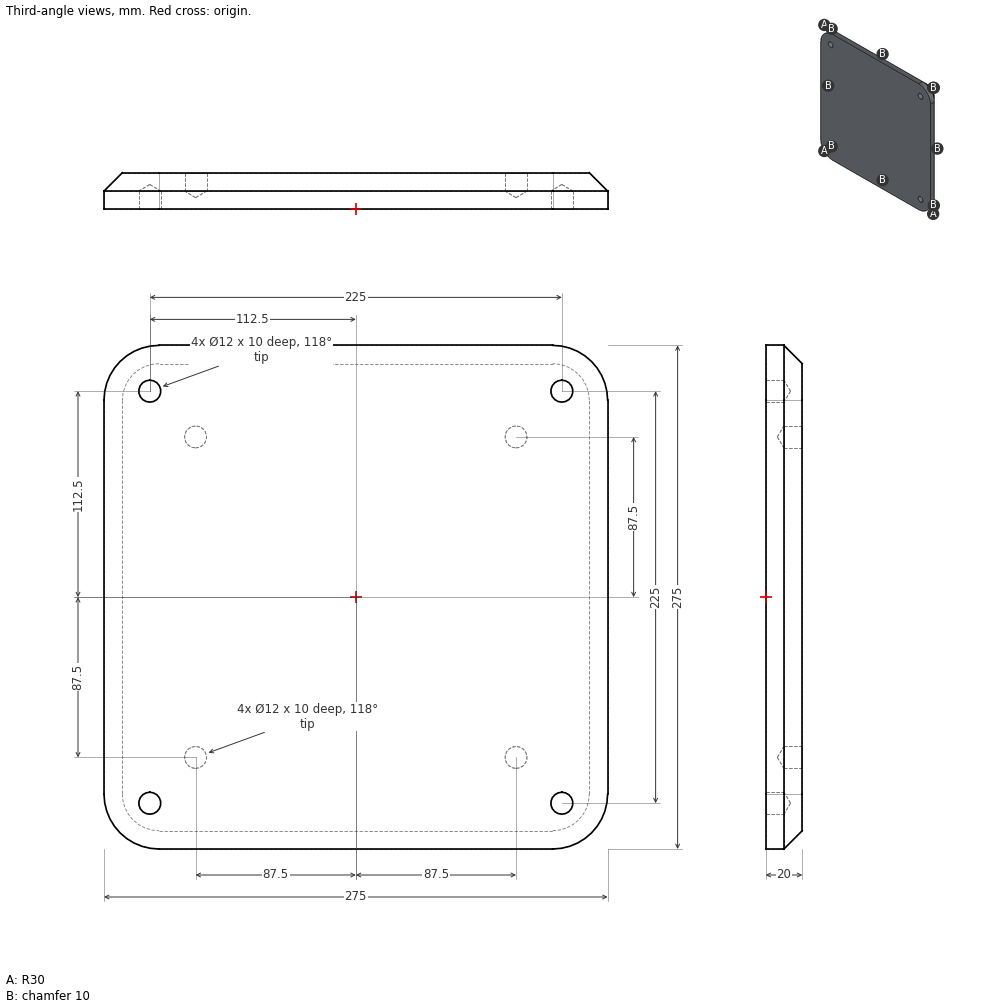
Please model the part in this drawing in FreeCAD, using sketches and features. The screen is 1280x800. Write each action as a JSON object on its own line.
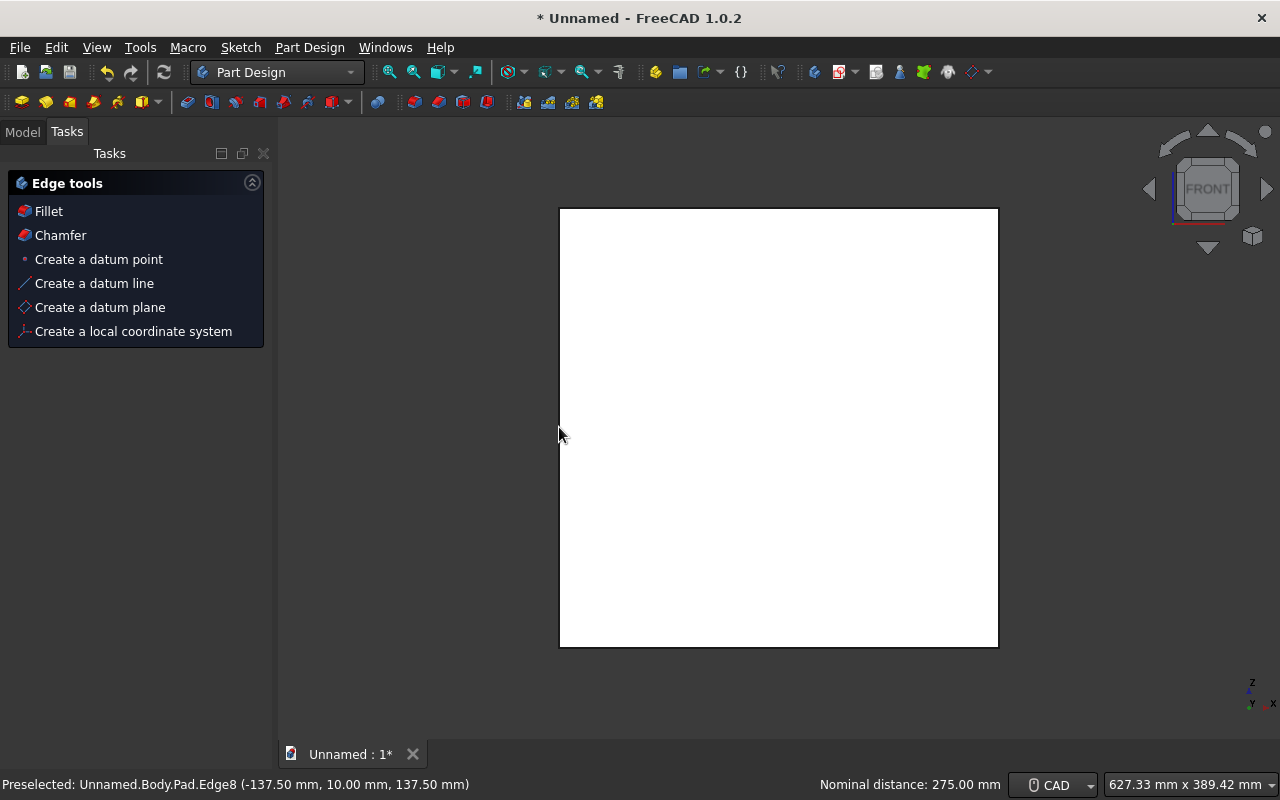
{"action": "key", "text": "3"}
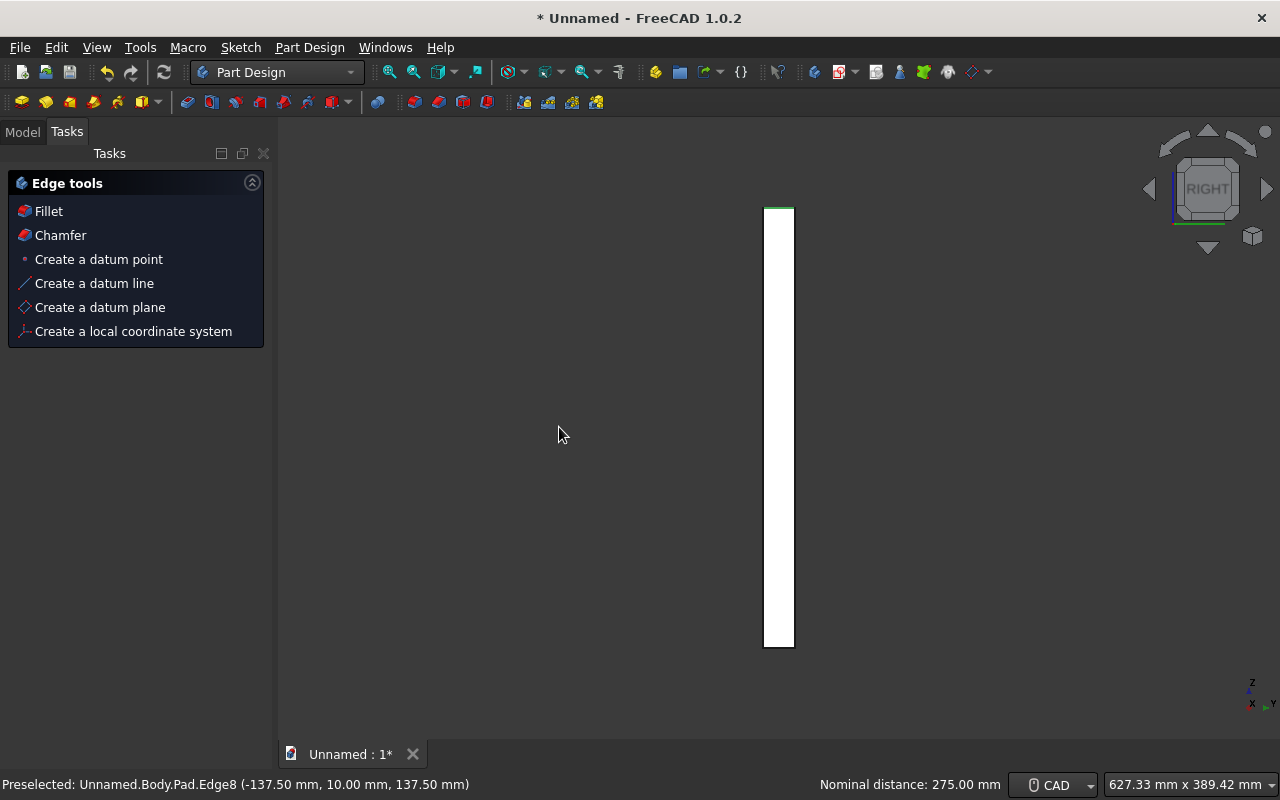
{"action": "left_click", "coordinate": [779, 647], "text": "ctrl"}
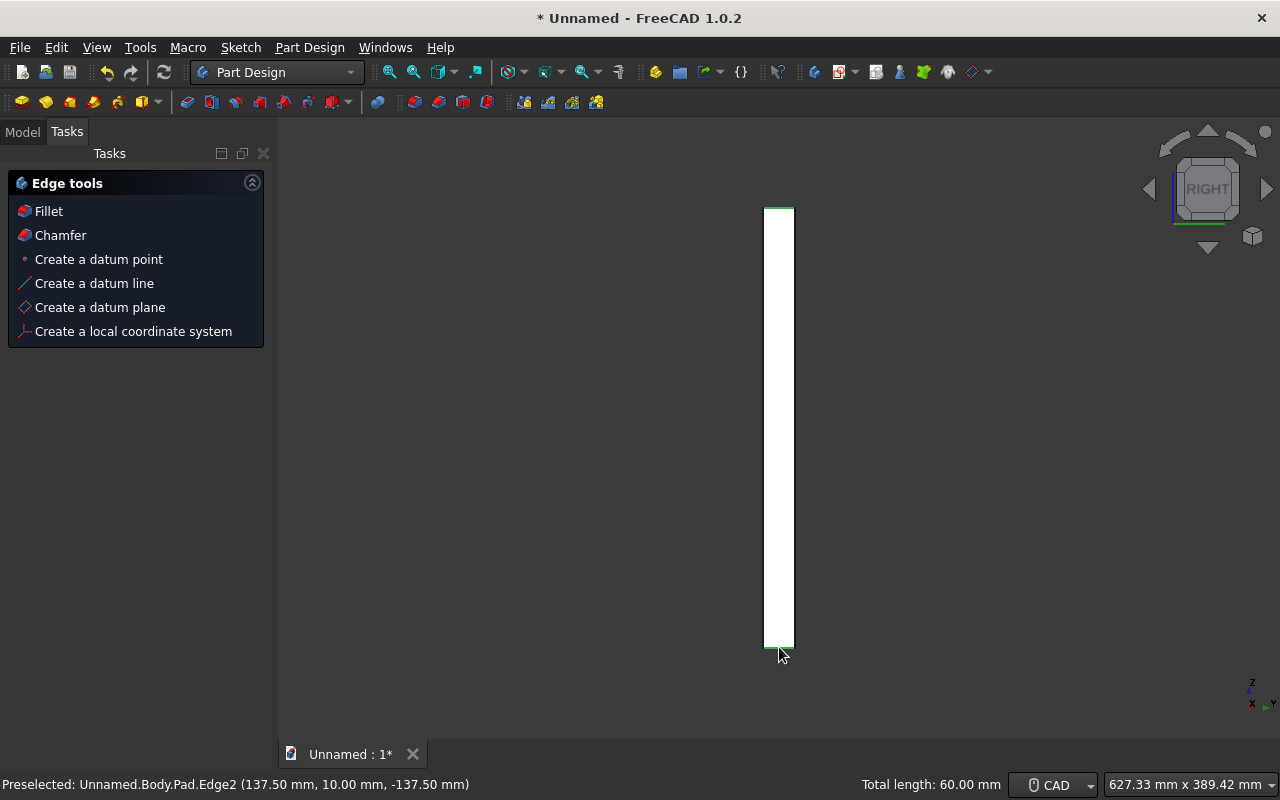
{"action": "key", "text": "5"}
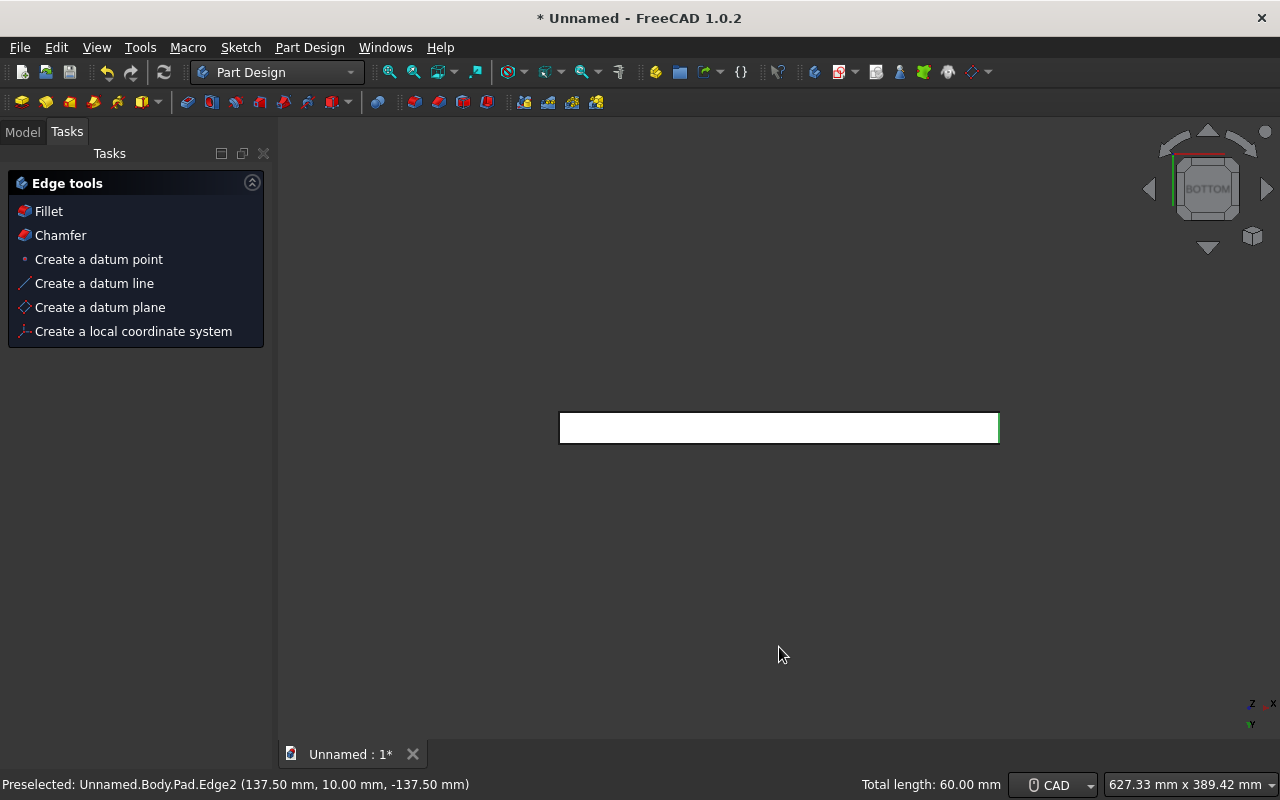
{"action": "key", "text": "v f"}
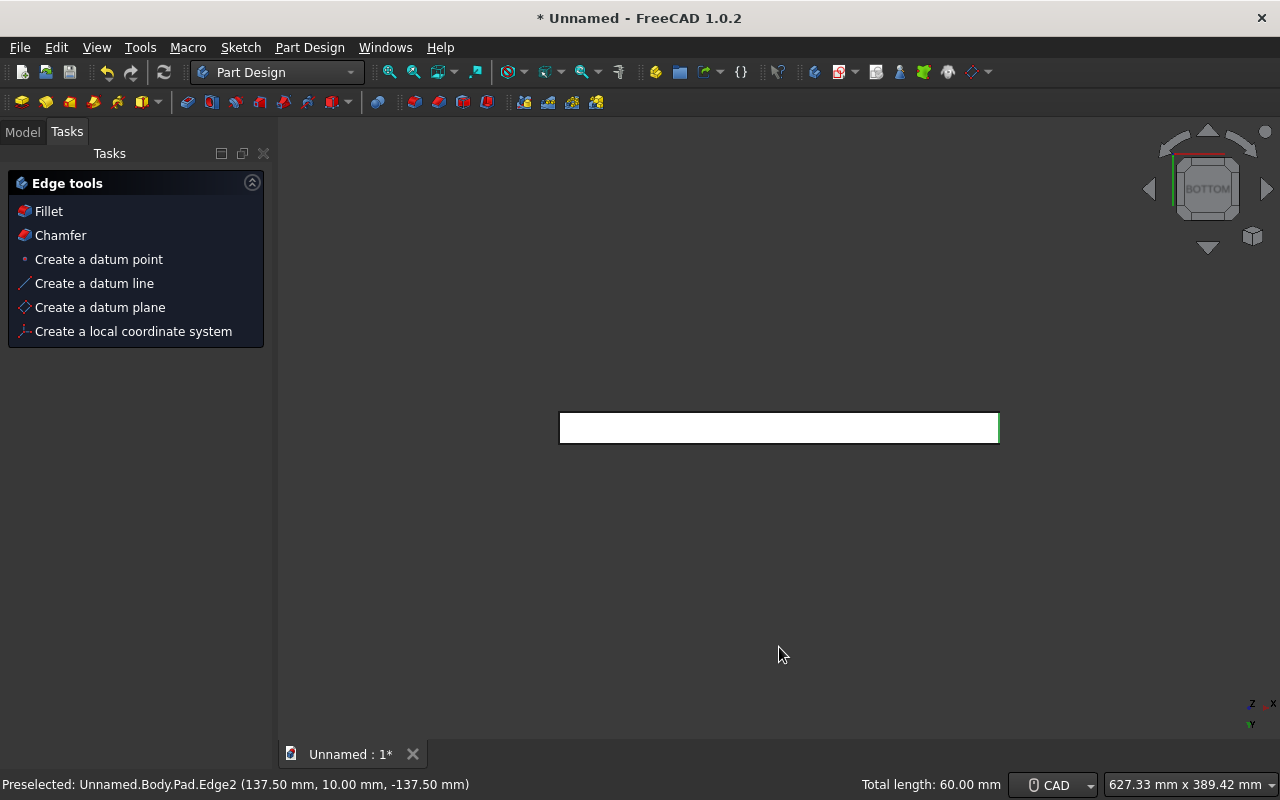
{"action": "left_click", "coordinate": [559, 427], "text": "ctrl"}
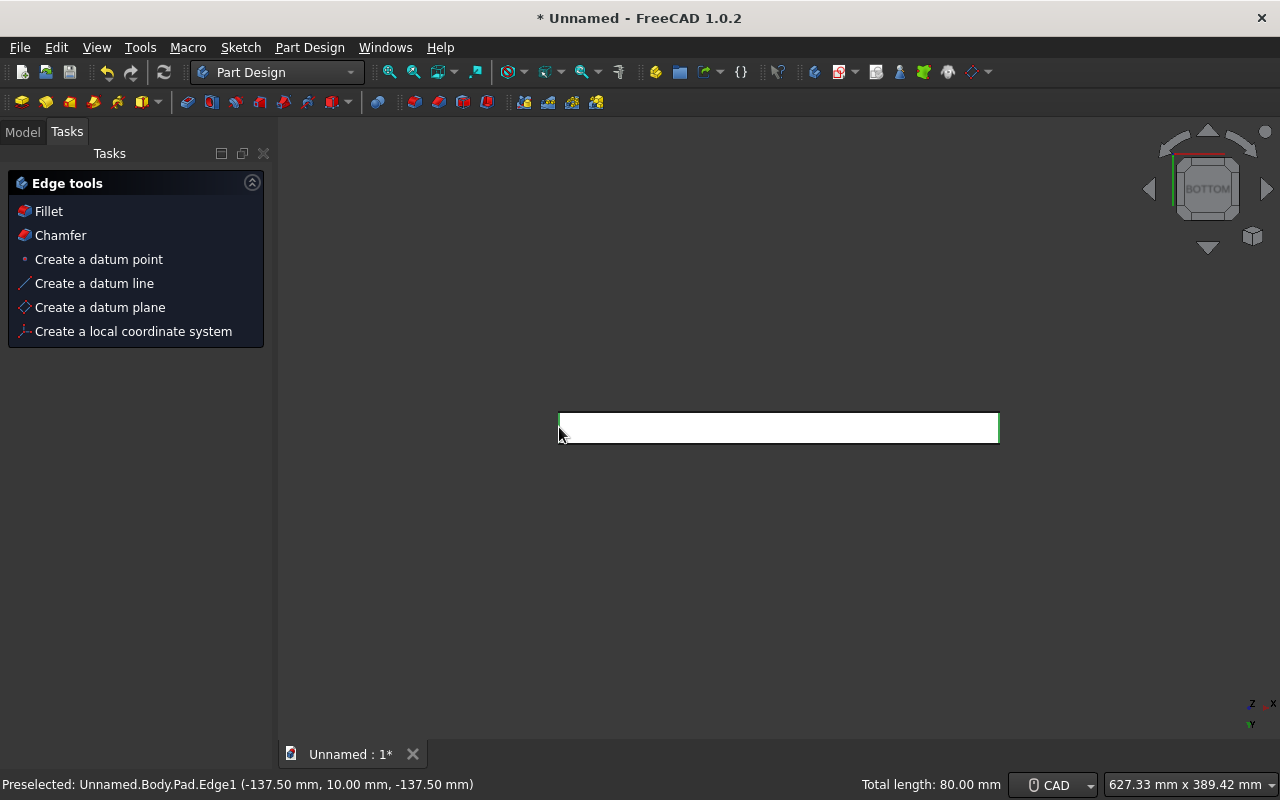
{"action": "left_click", "coordinate": [416, 102]}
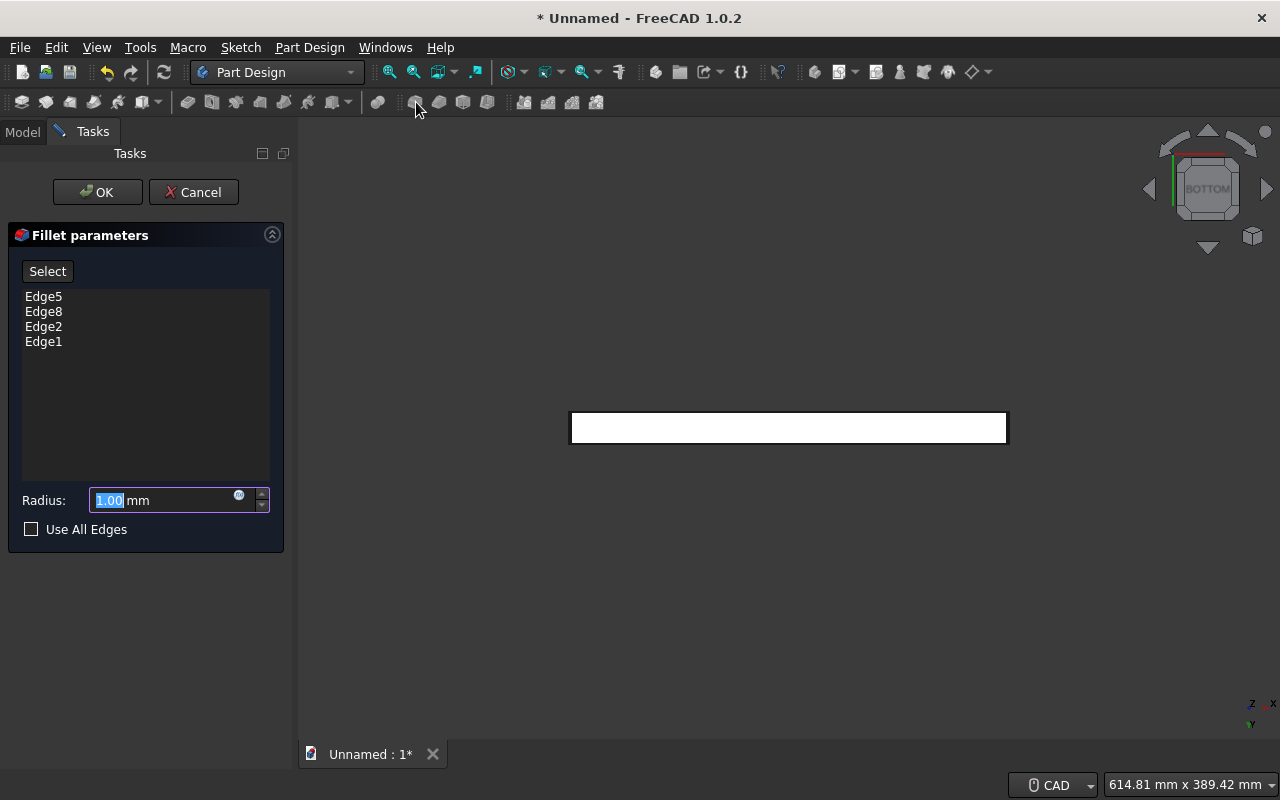
{"action": "type", "text": "30"}
{"action": "key", "text": "Tab"}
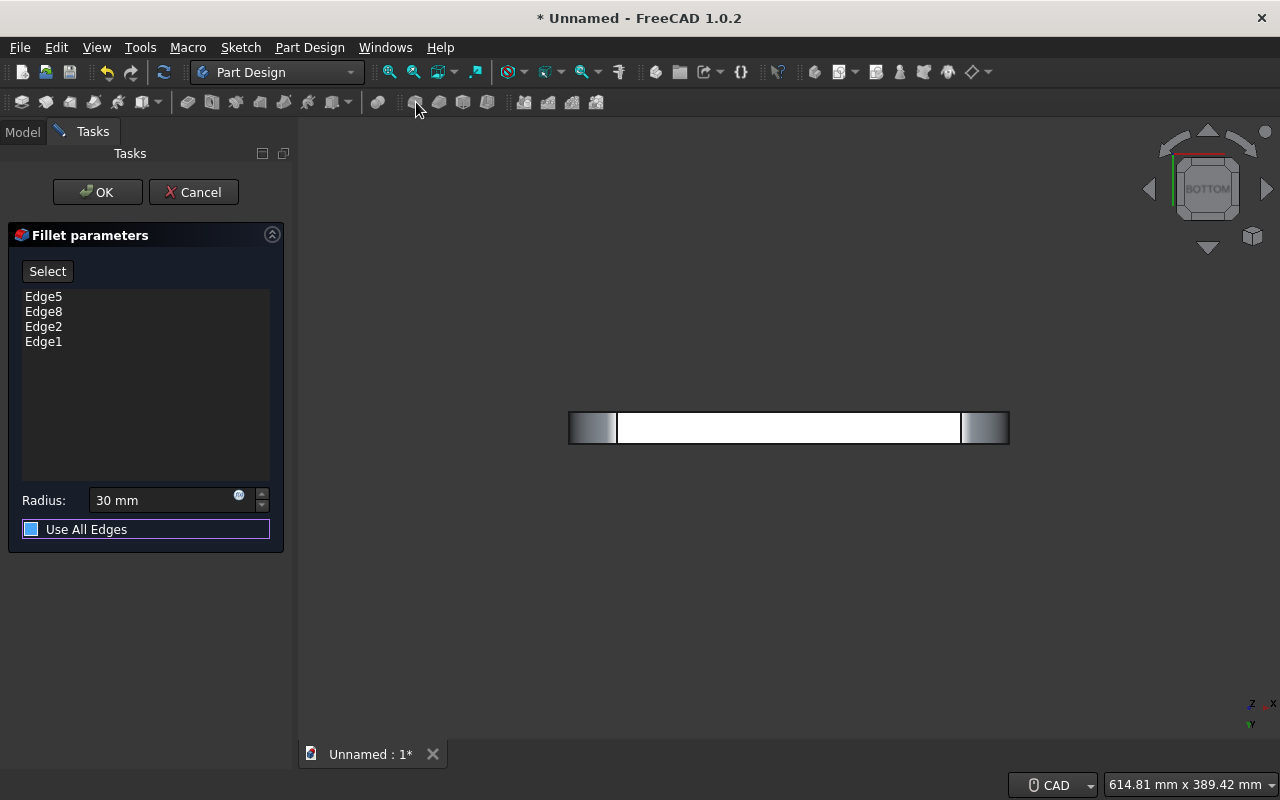
{"action": "left_click", "coordinate": [98, 192]}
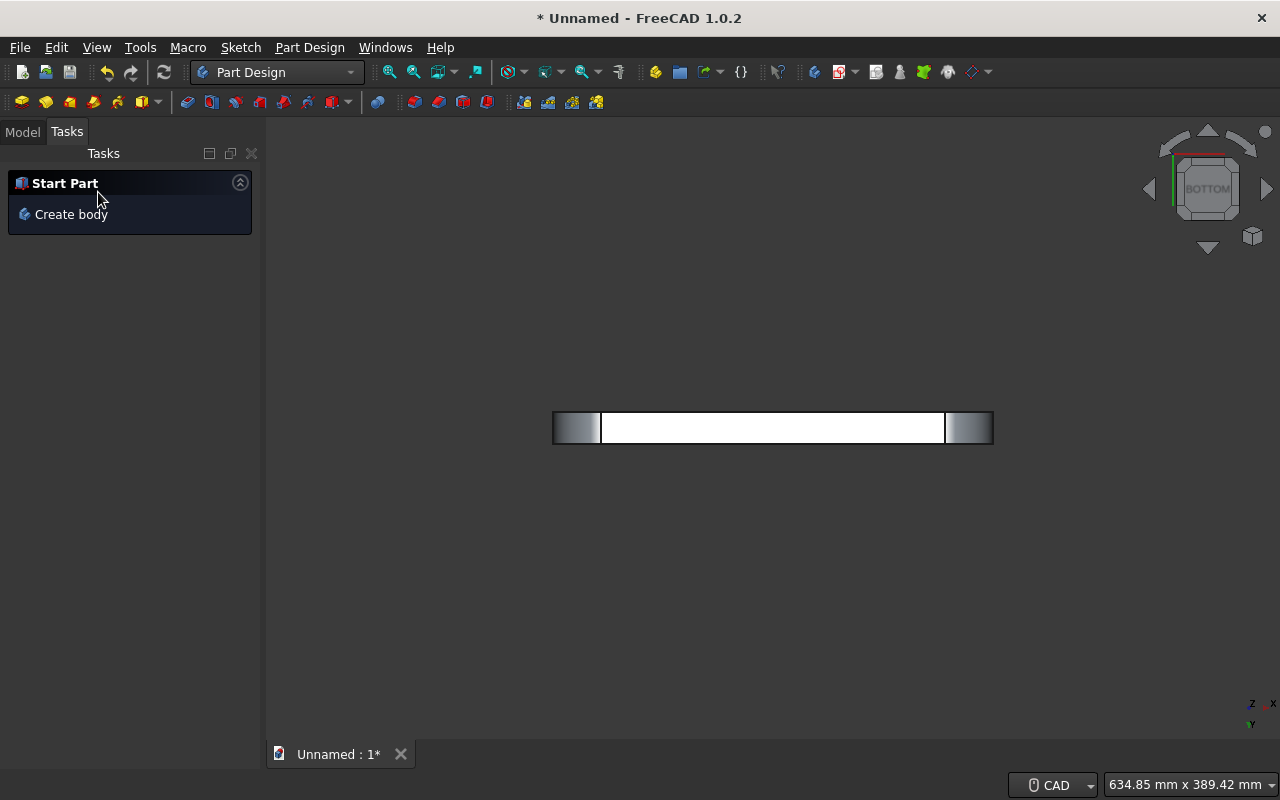
{"action": "key", "text": "v f"}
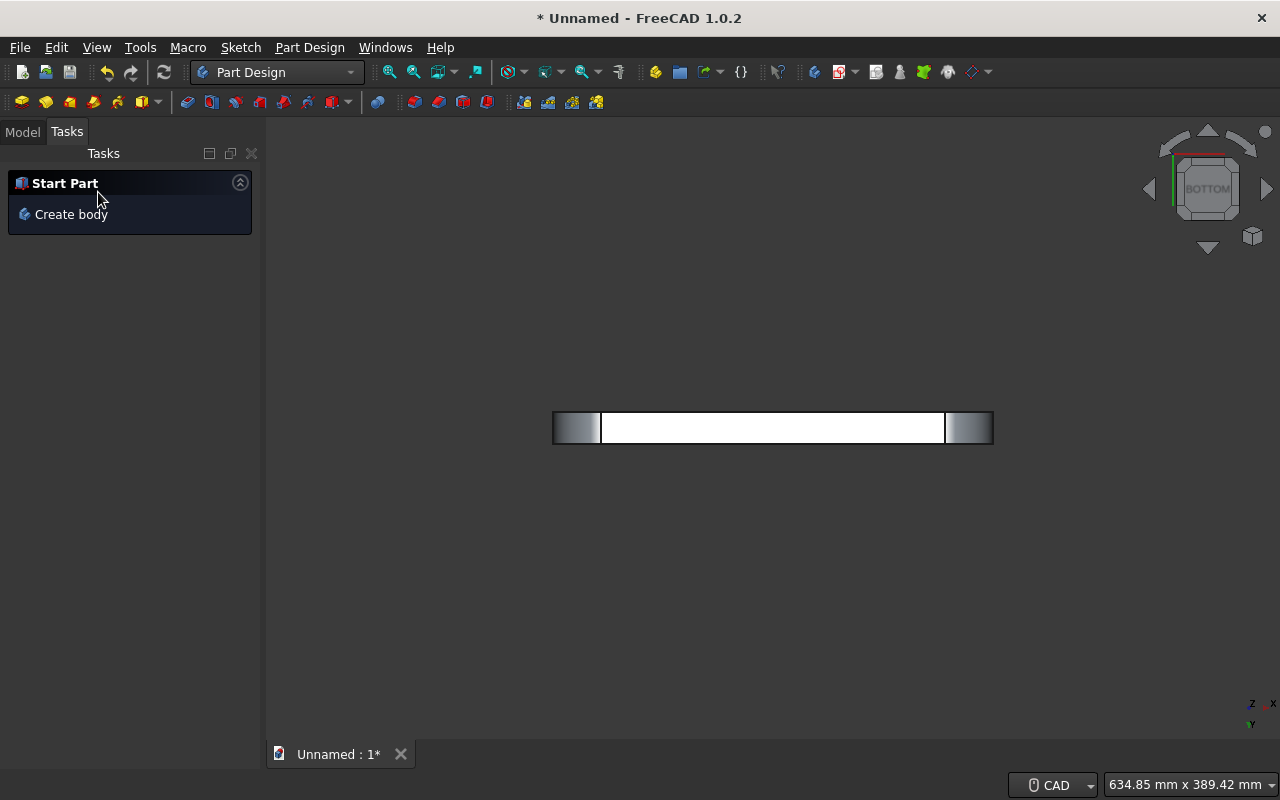
{"action": "key", "text": "0"}